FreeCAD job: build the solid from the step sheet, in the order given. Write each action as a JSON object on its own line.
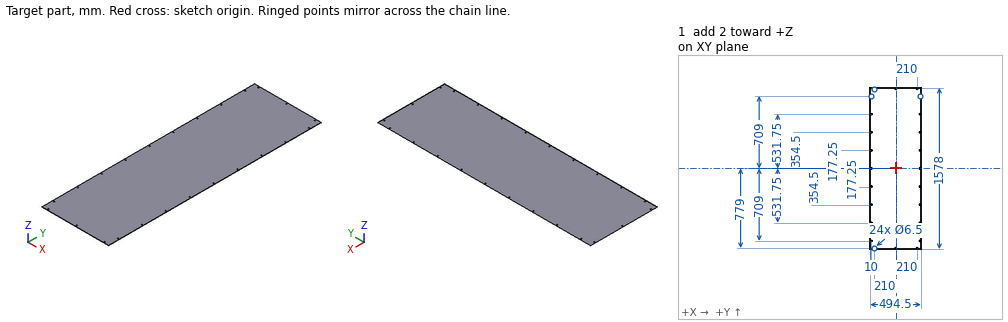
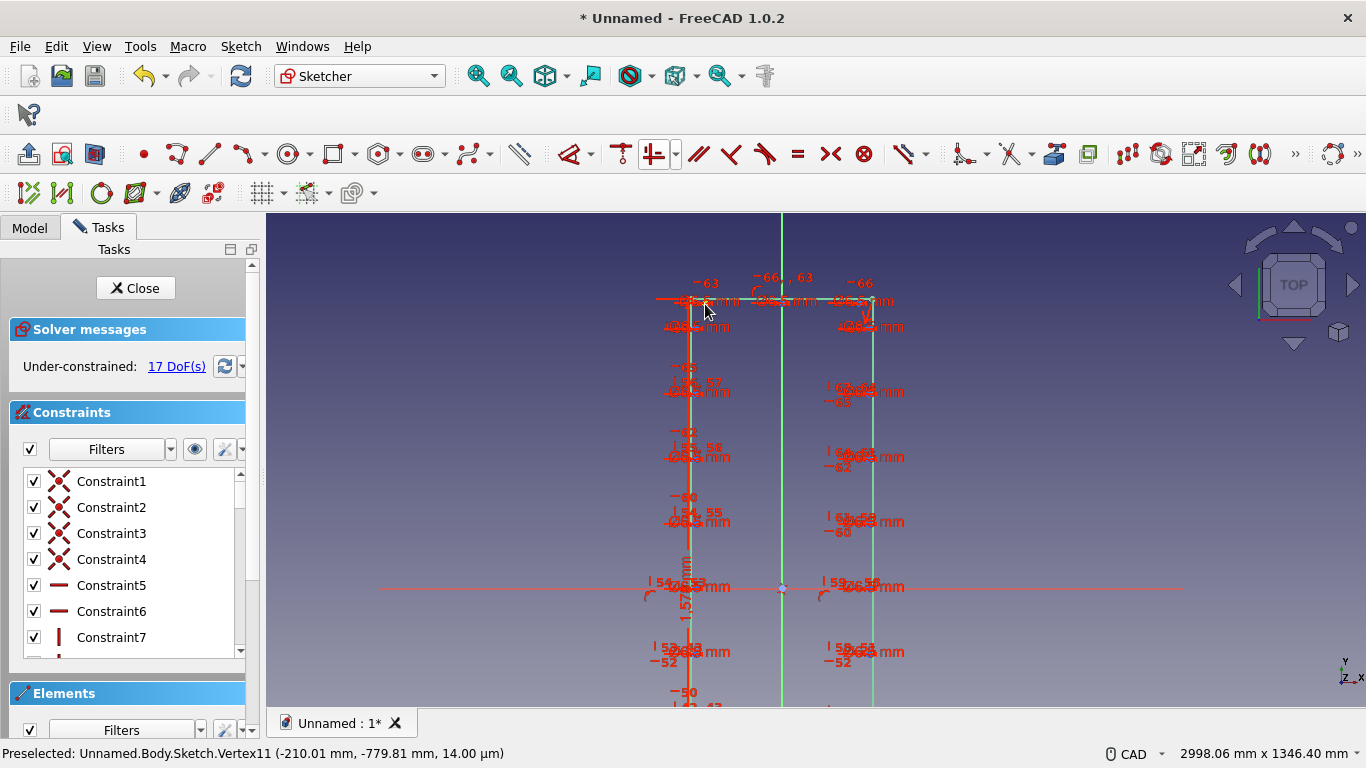
{"action": "left_click", "coordinate": [705, 303]}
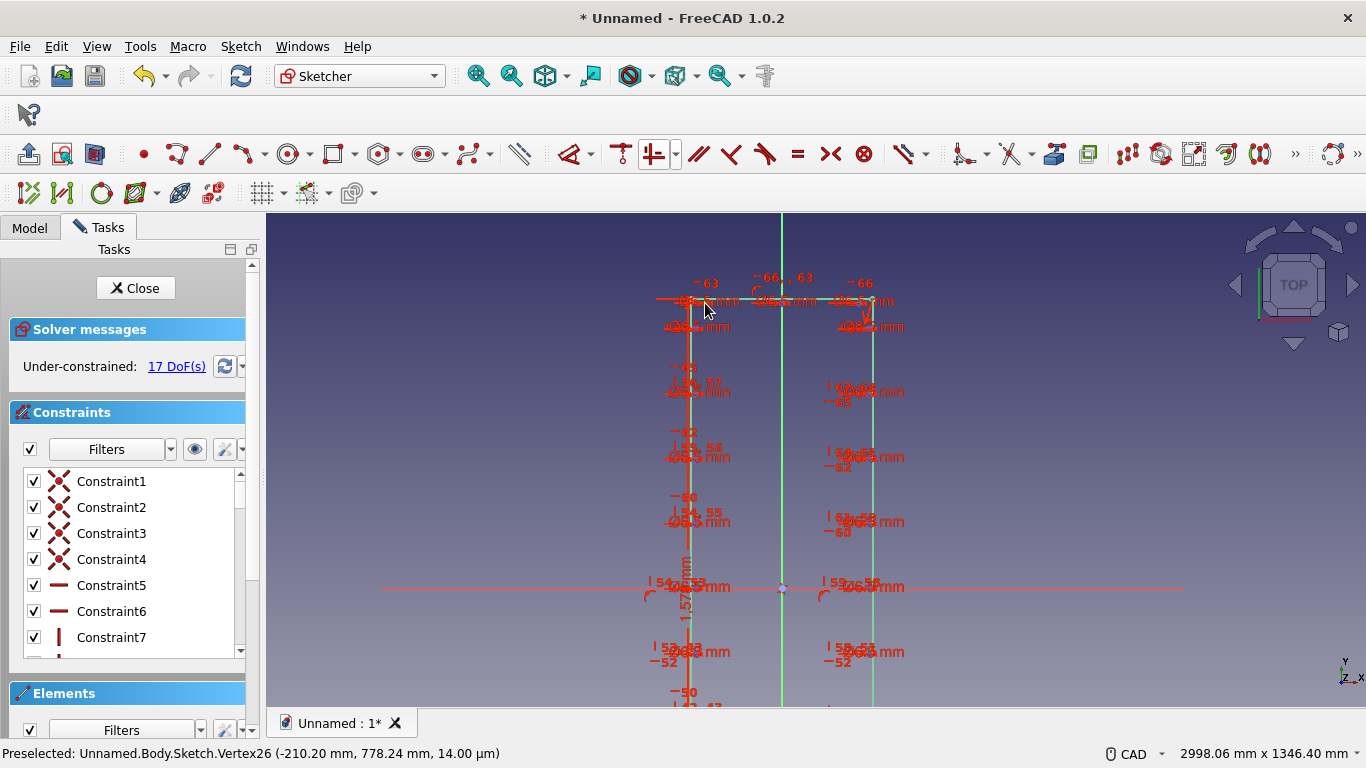
{"action": "left_click", "coordinate": [424, 589]}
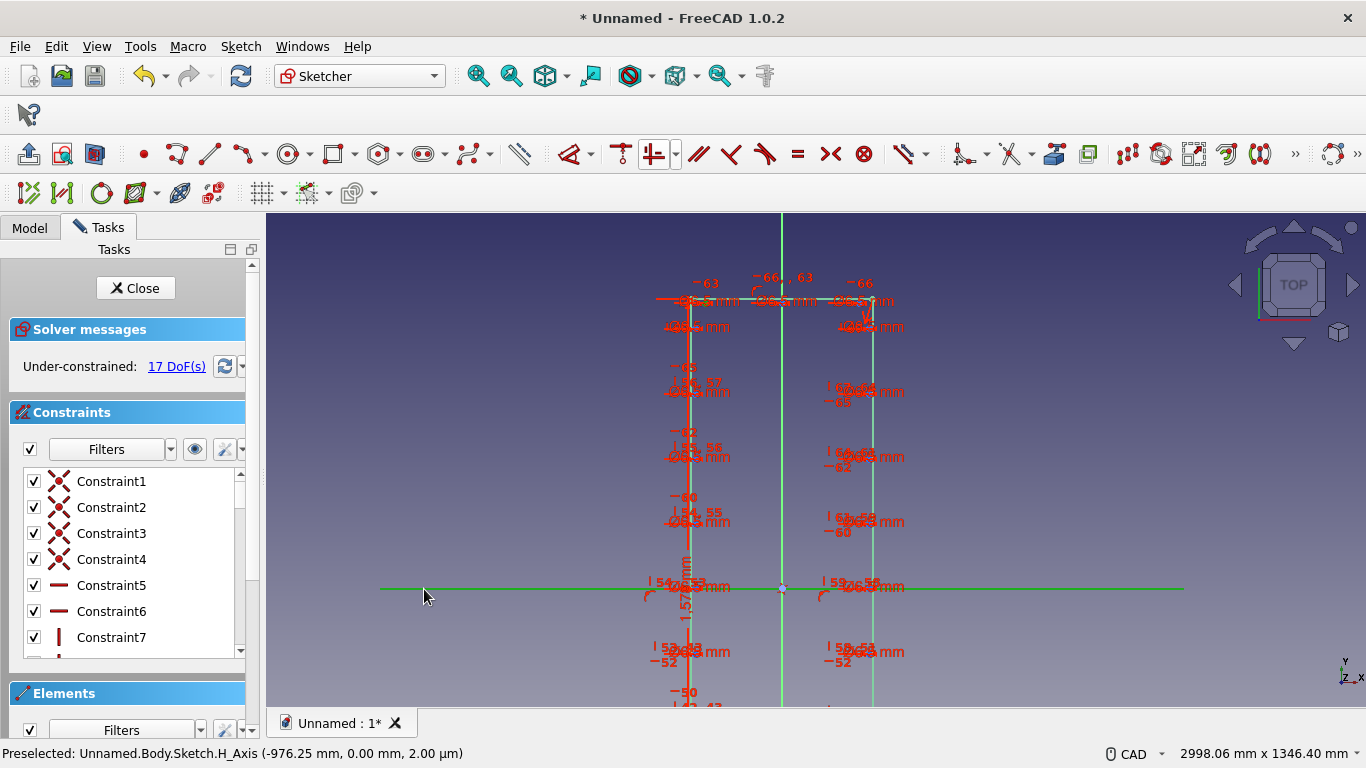
{"action": "left_click", "coordinate": [831, 154]}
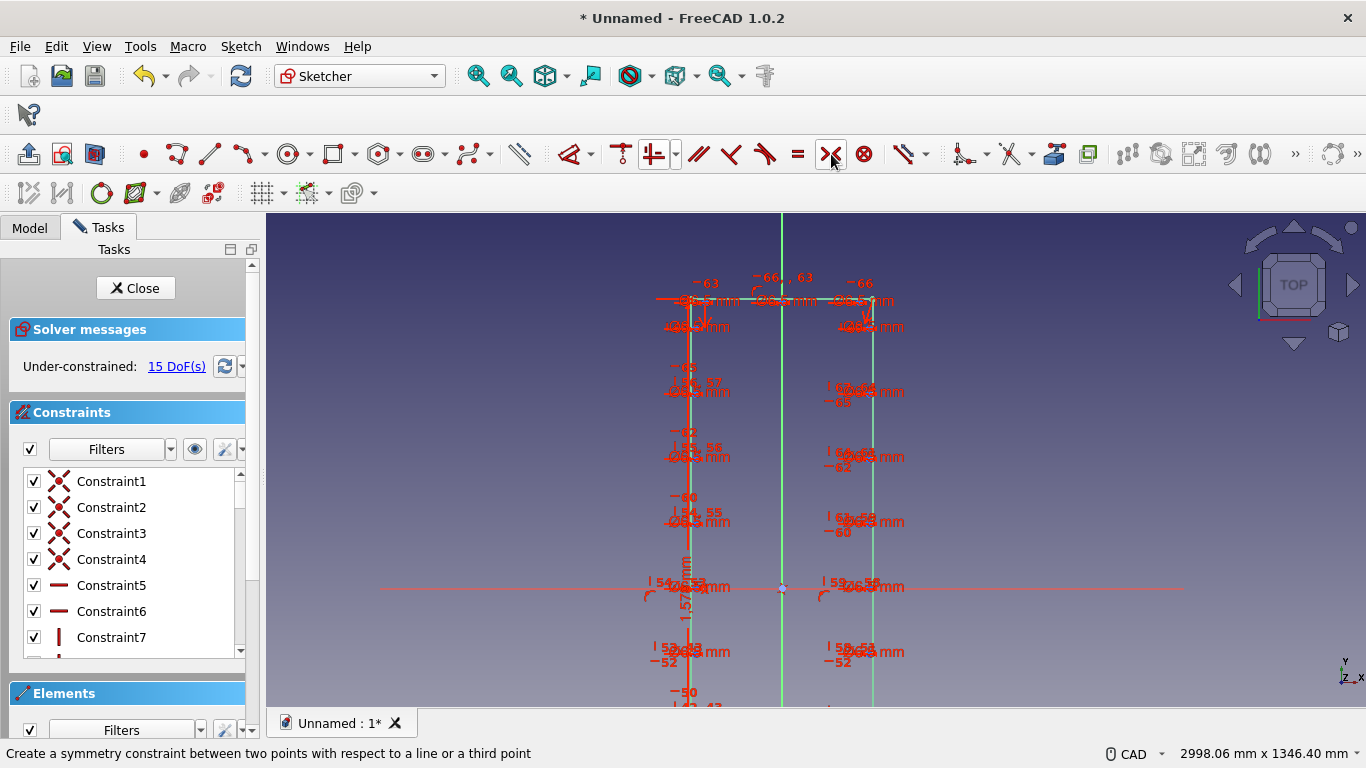
{"action": "left_click", "coordinate": [695, 329]}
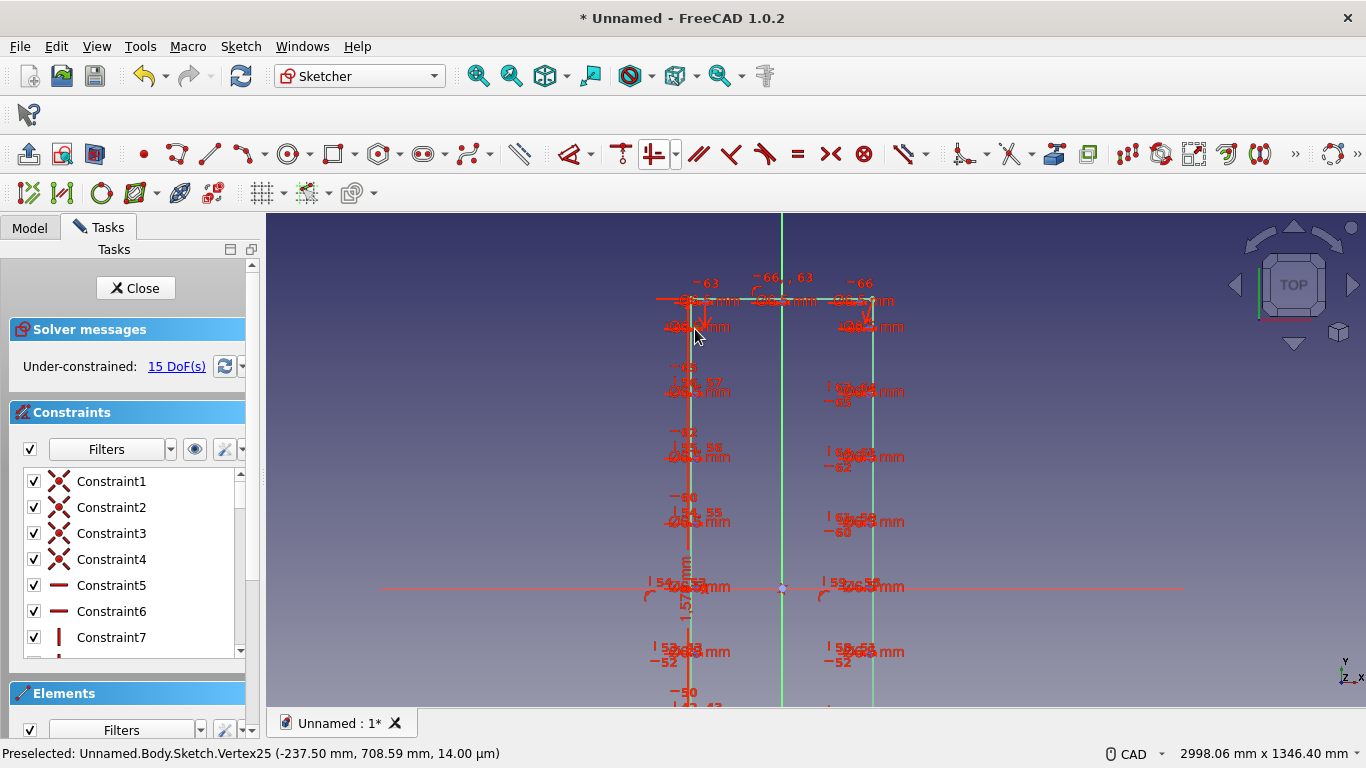
{"action": "left_click", "coordinate": [869, 329]}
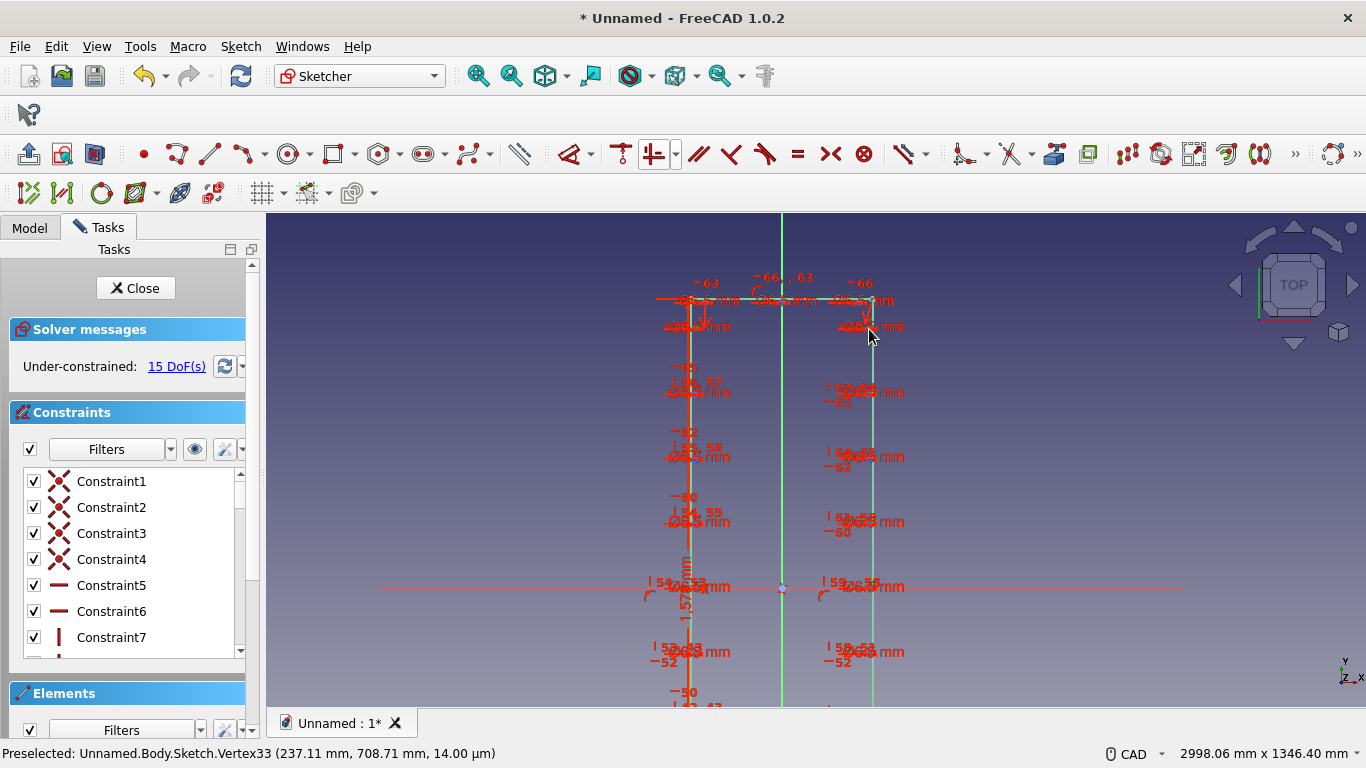
{"action": "left_click", "coordinate": [782, 648]}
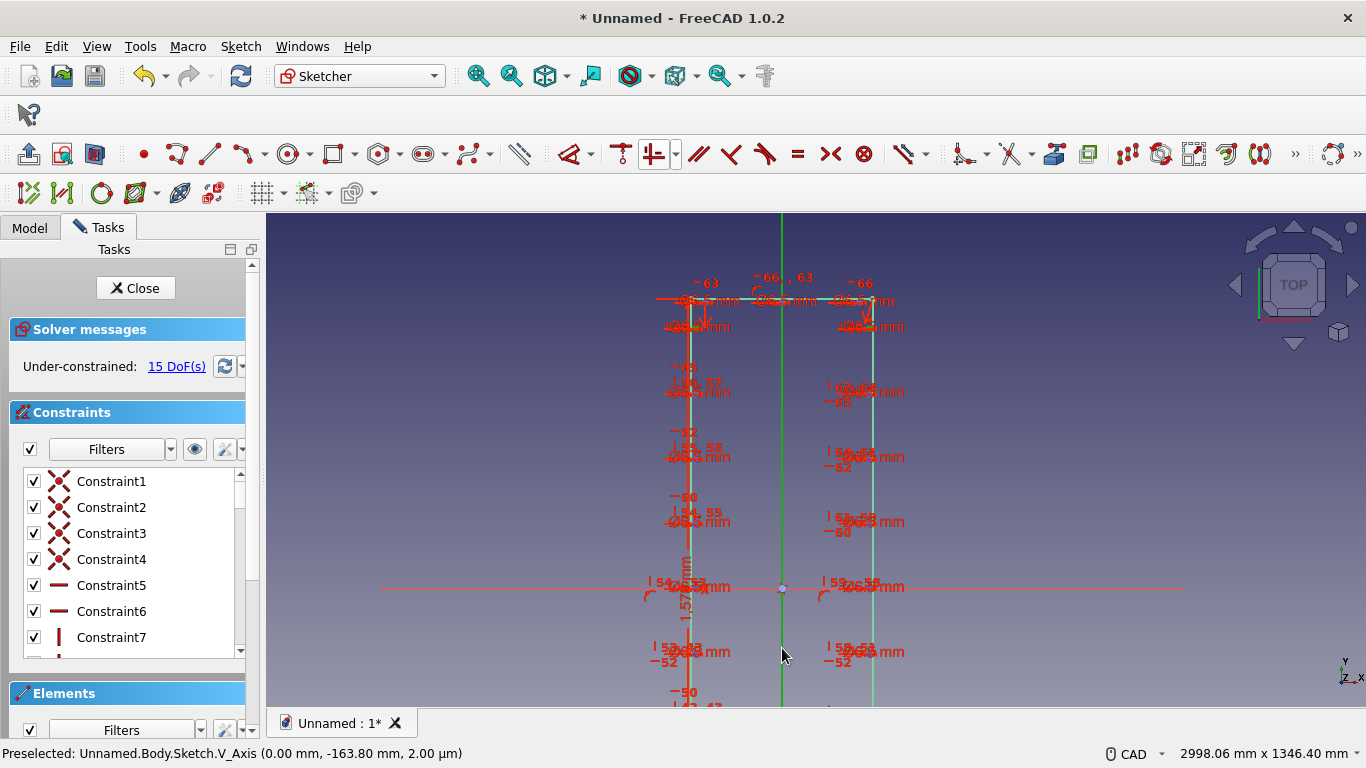
{"action": "key", "text": "s"}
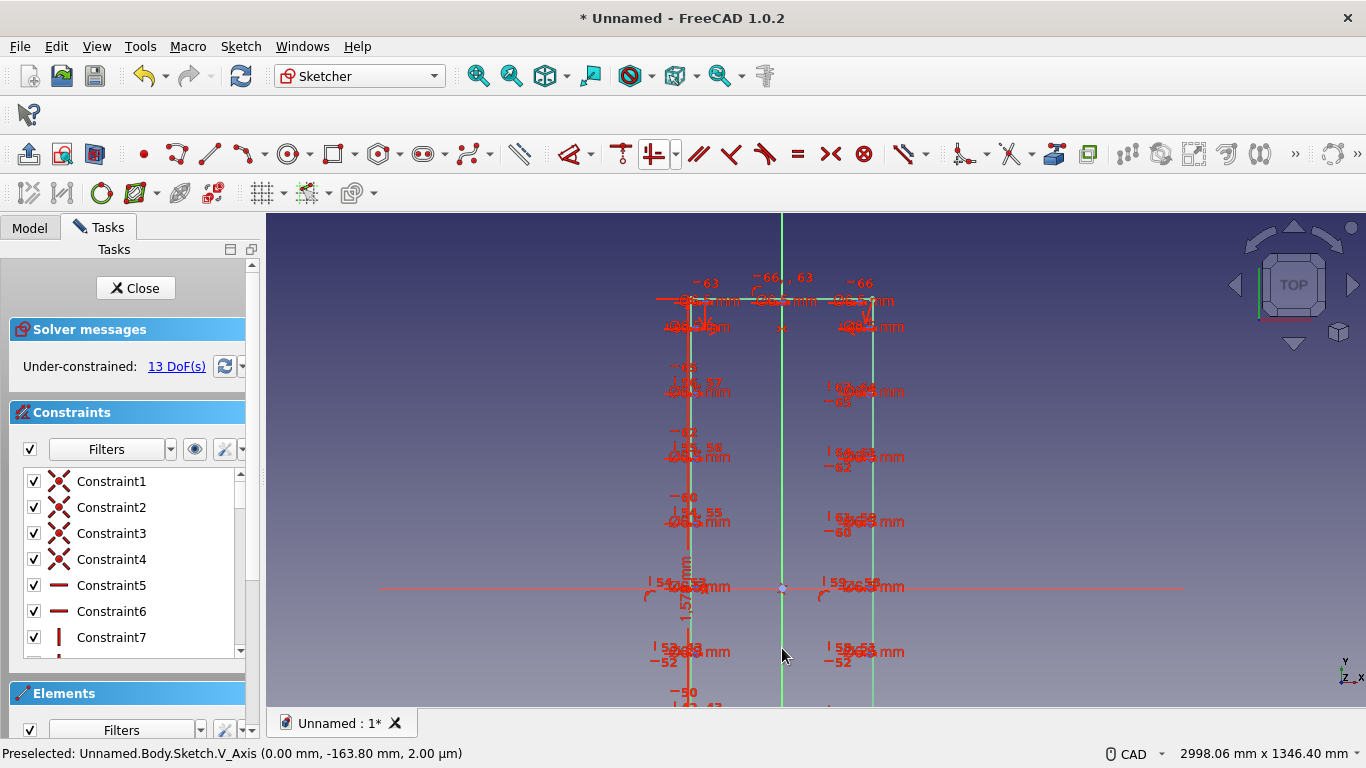
{"action": "key", "text": "d"}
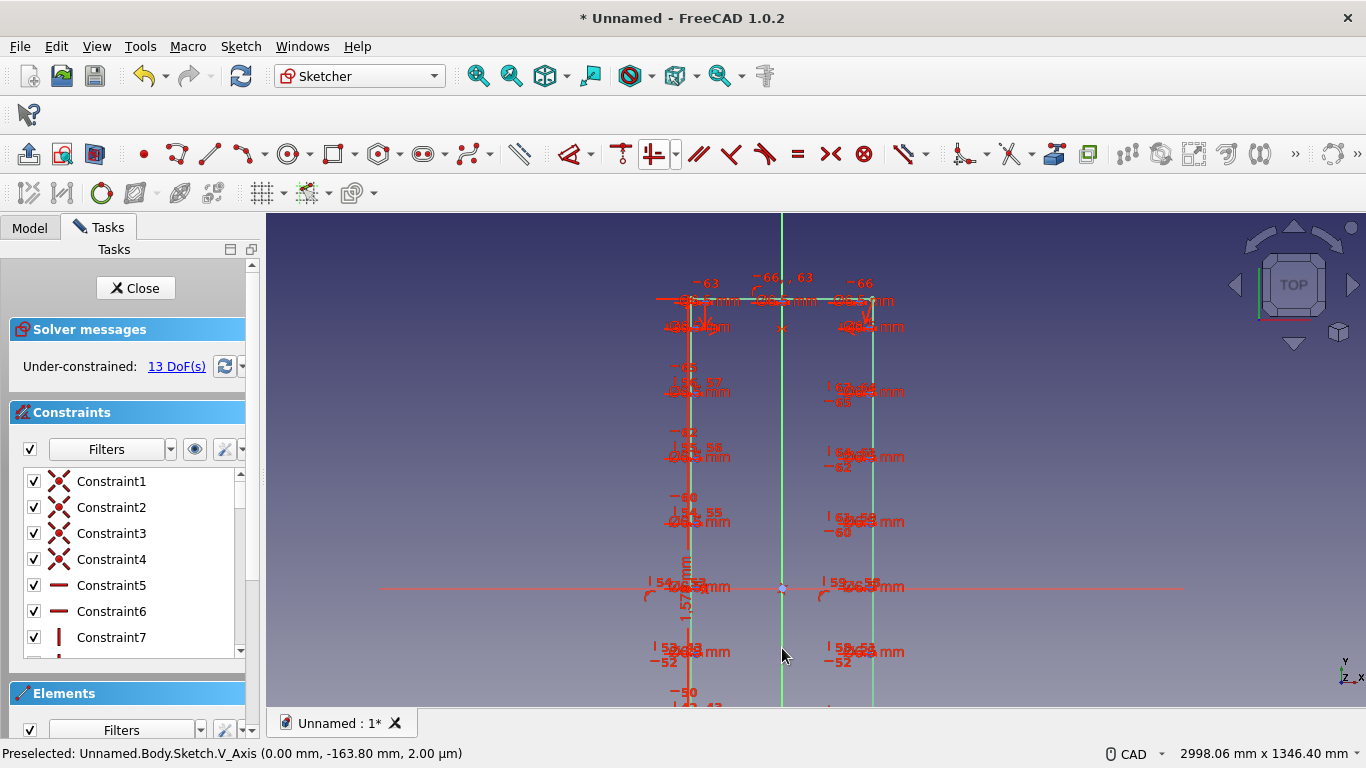
{"action": "scroll", "coordinate": [705, 303], "scroll_direction": "down", "scroll_amount": 3}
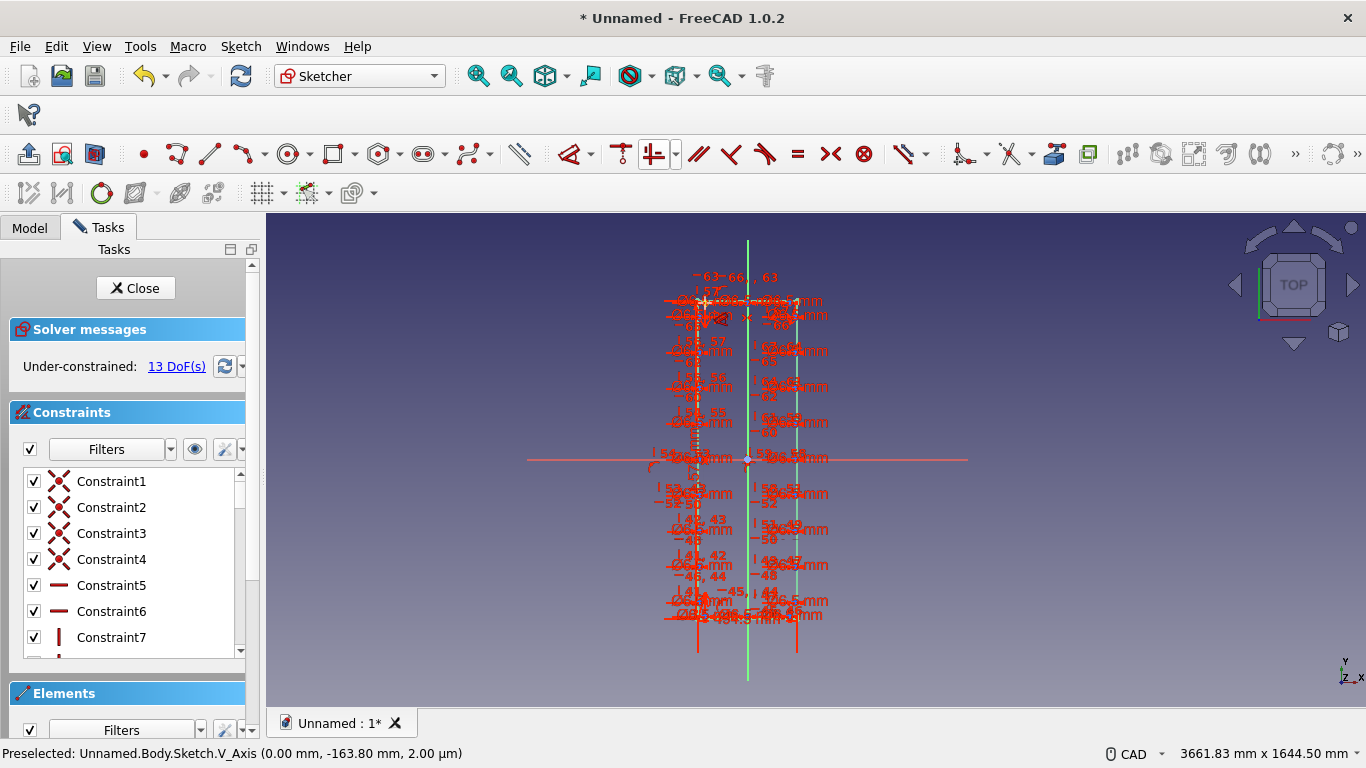
{"action": "left_click", "coordinate": [700, 603]}
{"action": "left_click", "coordinate": [666, 531]}